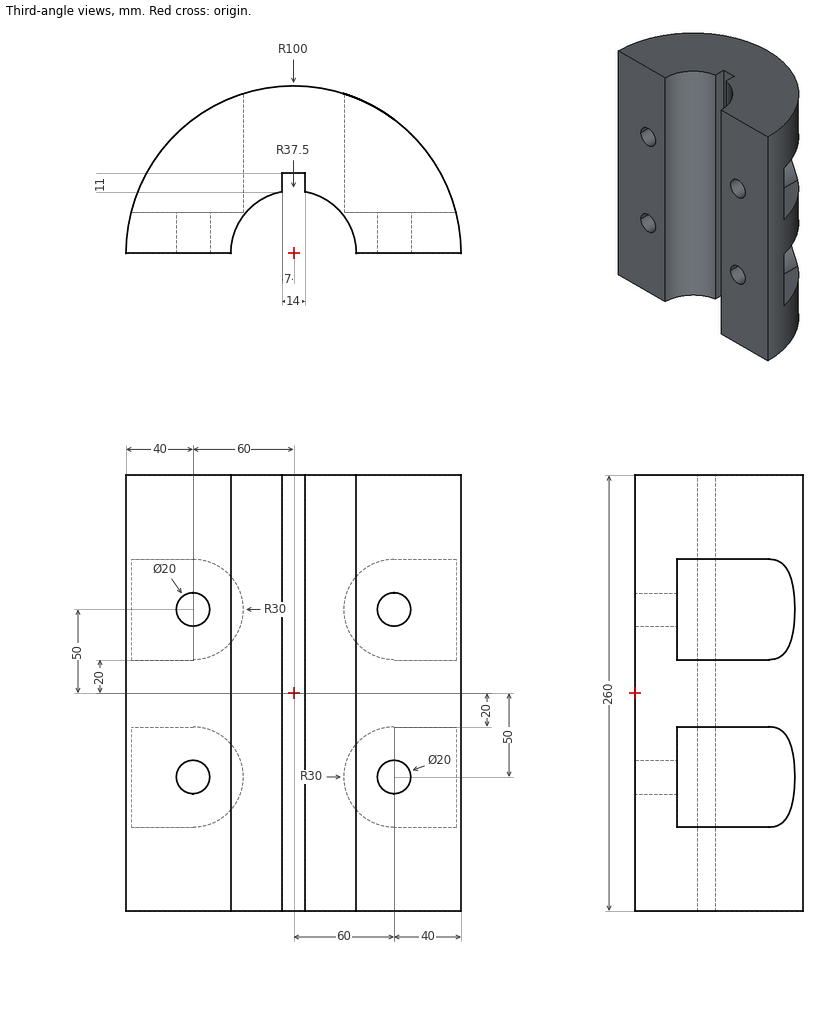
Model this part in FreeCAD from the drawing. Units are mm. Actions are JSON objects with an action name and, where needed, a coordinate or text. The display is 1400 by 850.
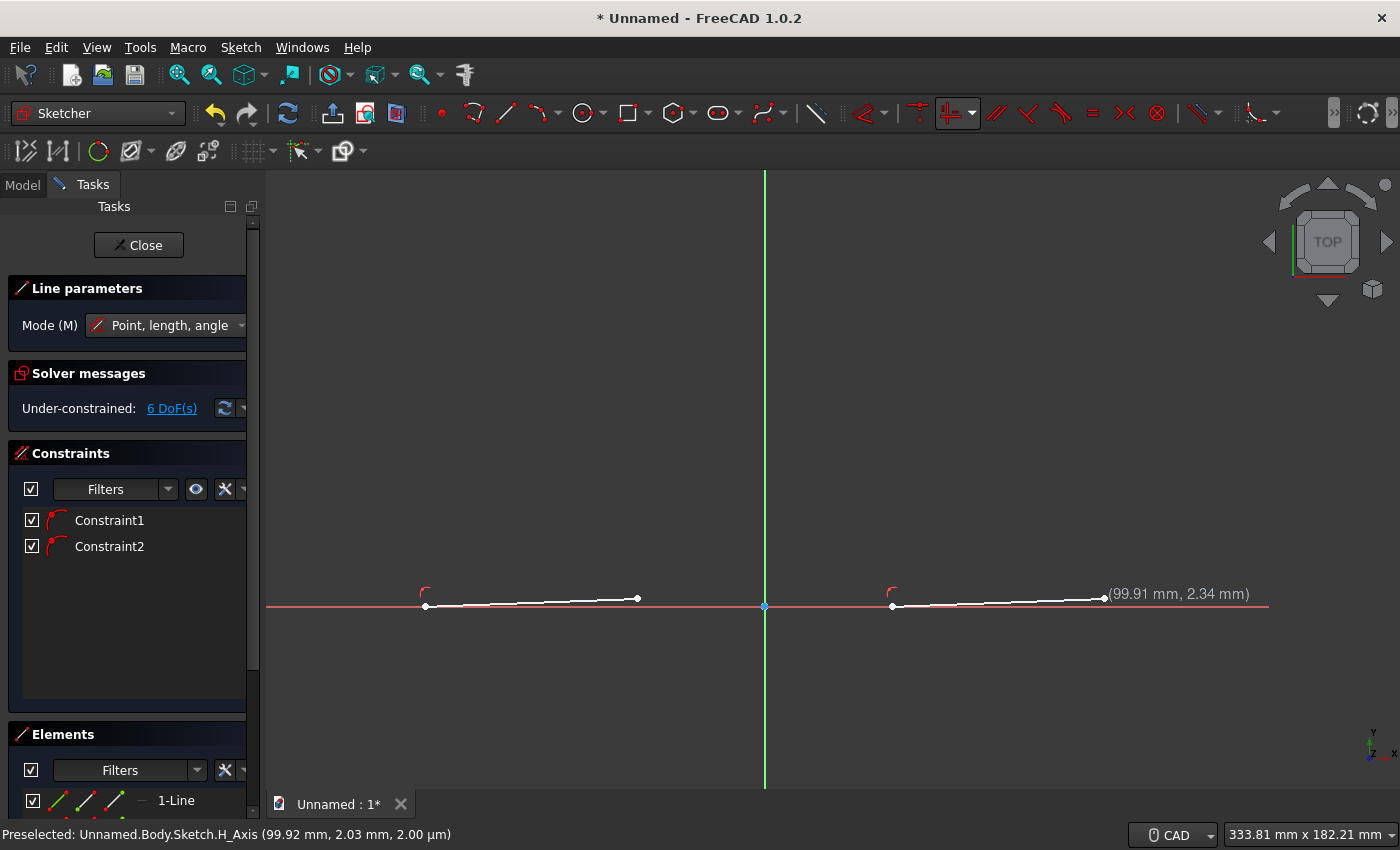
{"action": "left_click", "coordinate": [538, 114]}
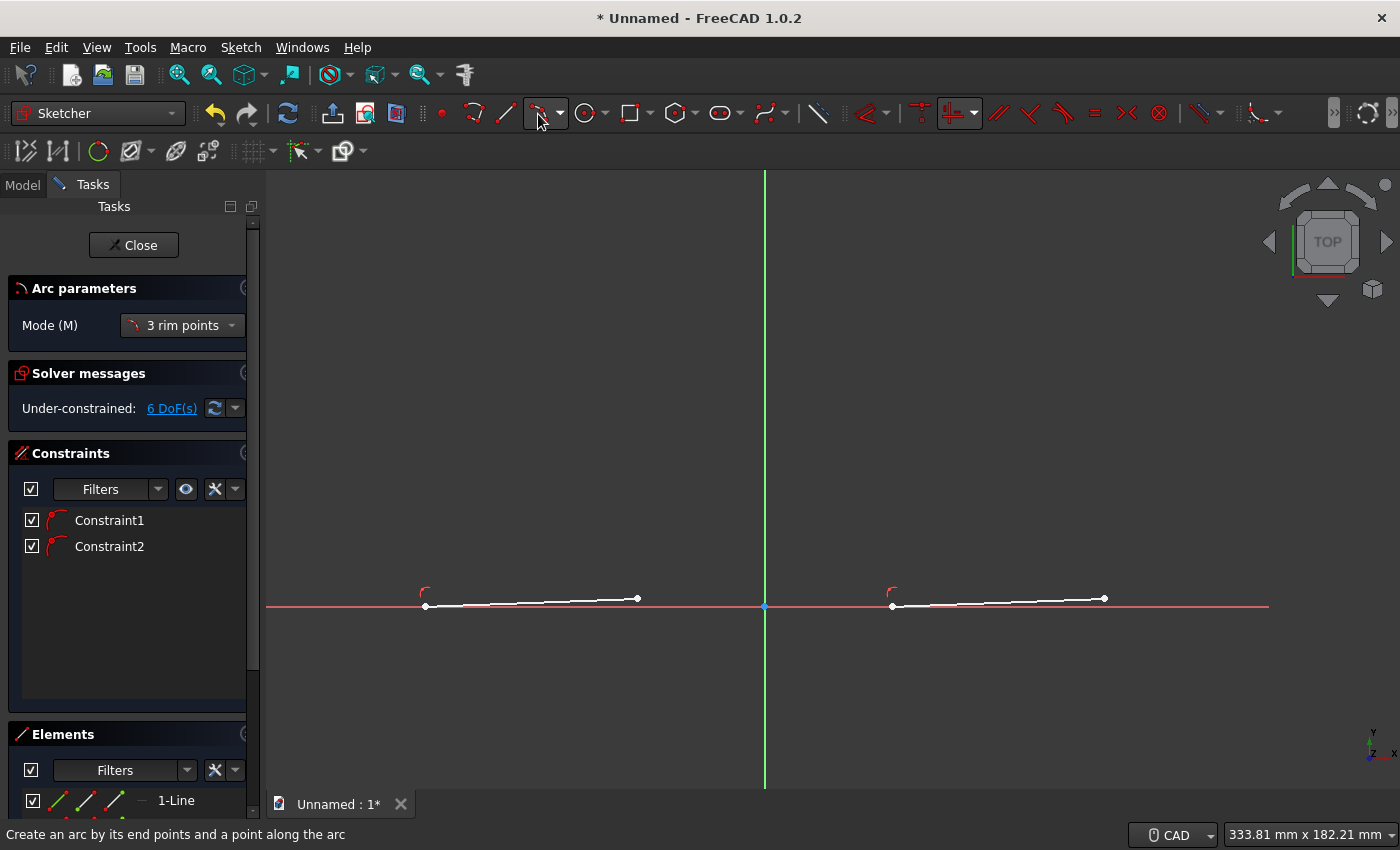
{"action": "left_click", "coordinate": [637, 599]}
{"action": "left_click", "coordinate": [892, 607]}
{"action": "left_click", "coordinate": [804, 486]}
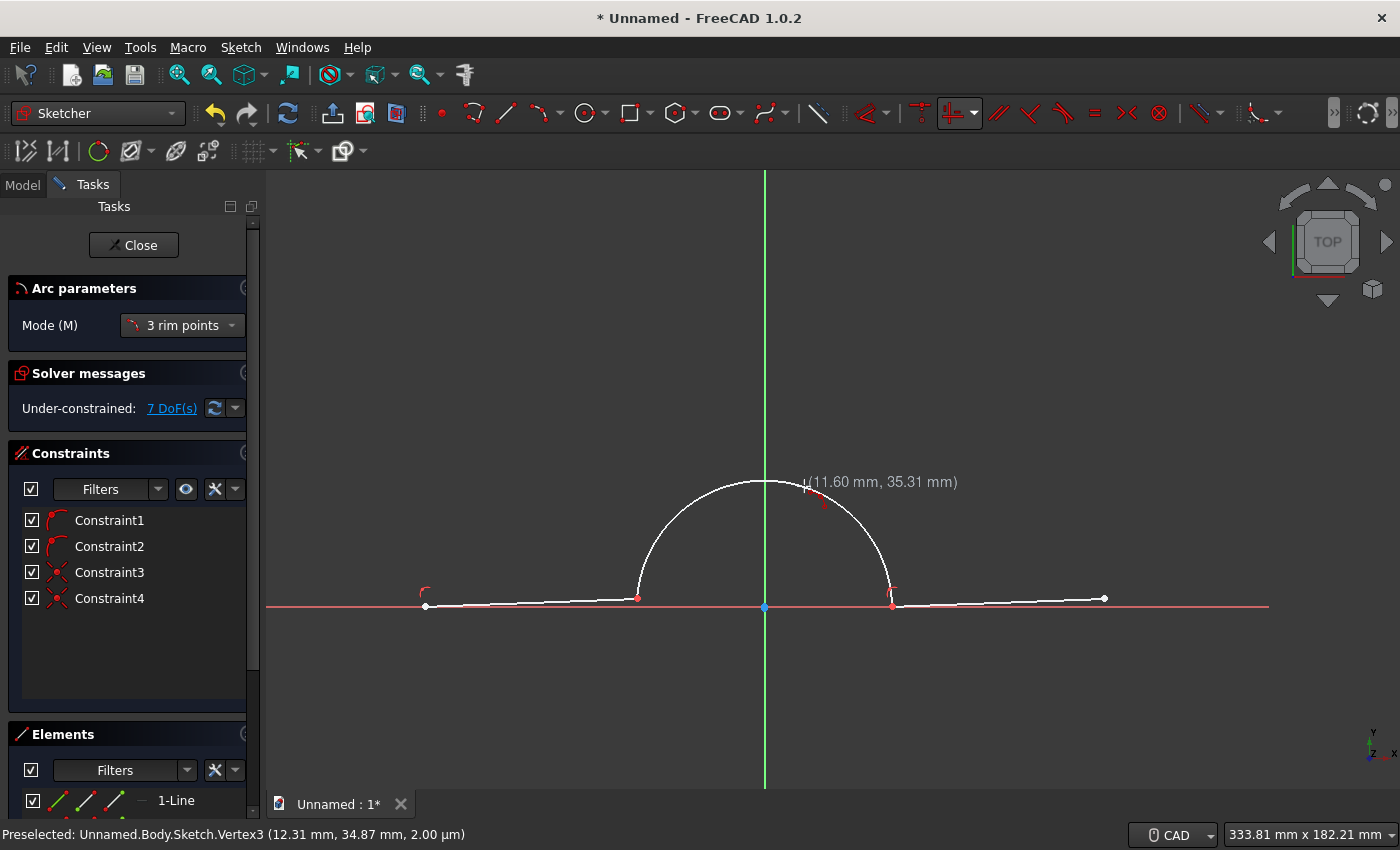
{"action": "left_click", "coordinate": [1104, 599]}
{"action": "left_click", "coordinate": [425, 607]}
{"action": "left_click", "coordinate": [870, 284]}
{"action": "key", "text": "Escape"}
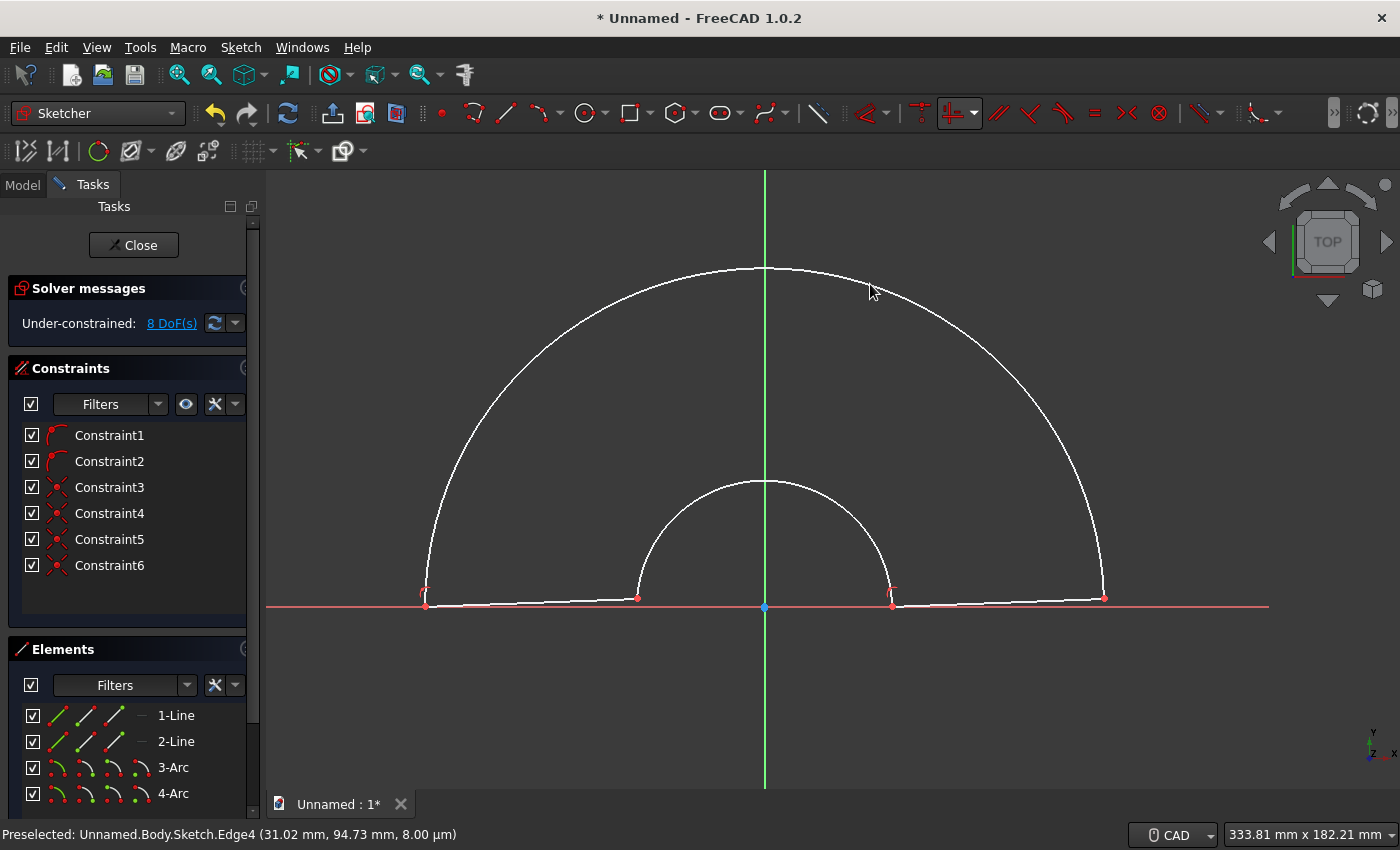
{"action": "left_click", "coordinate": [489, 605]}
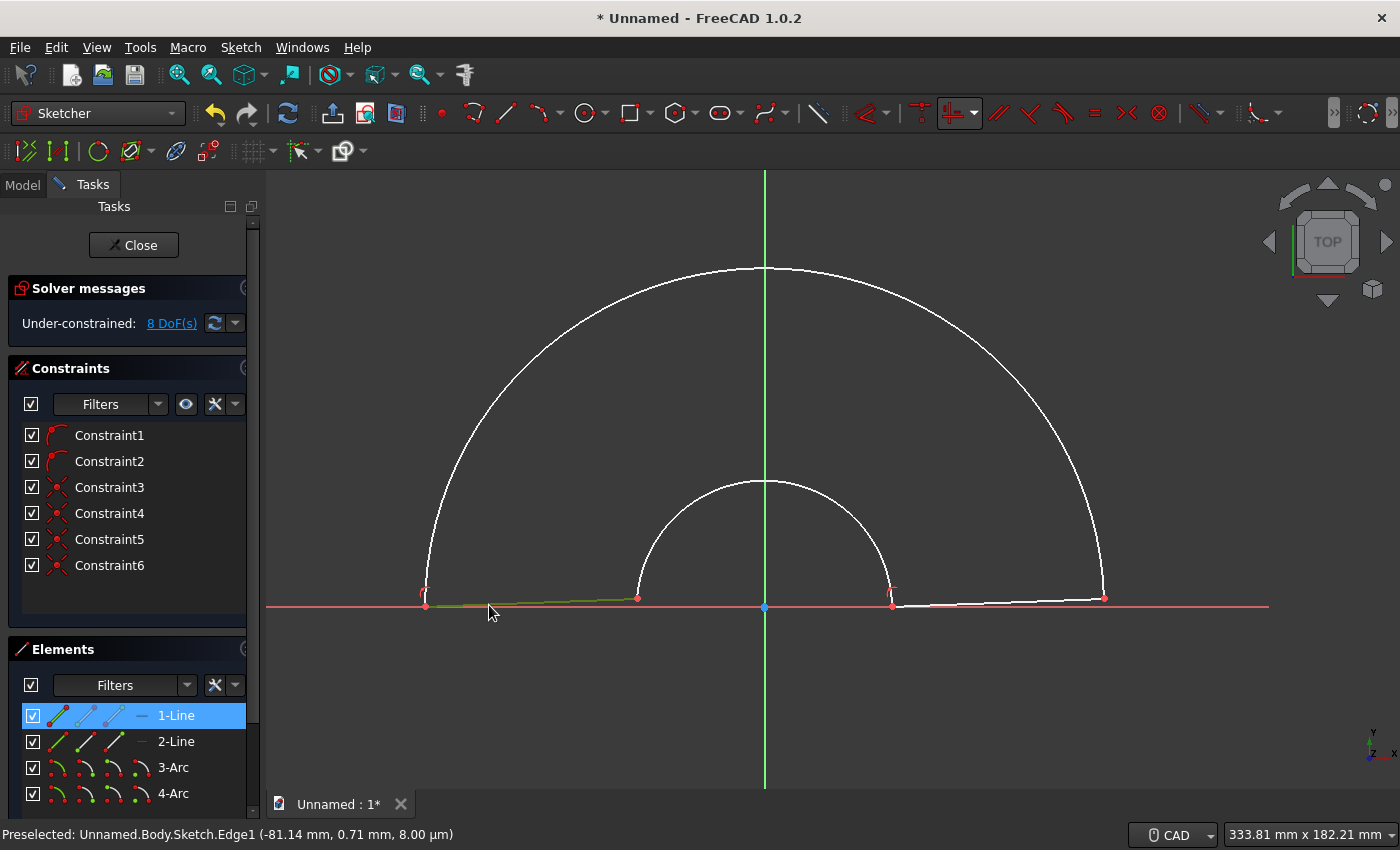
{"action": "key", "text": "h"}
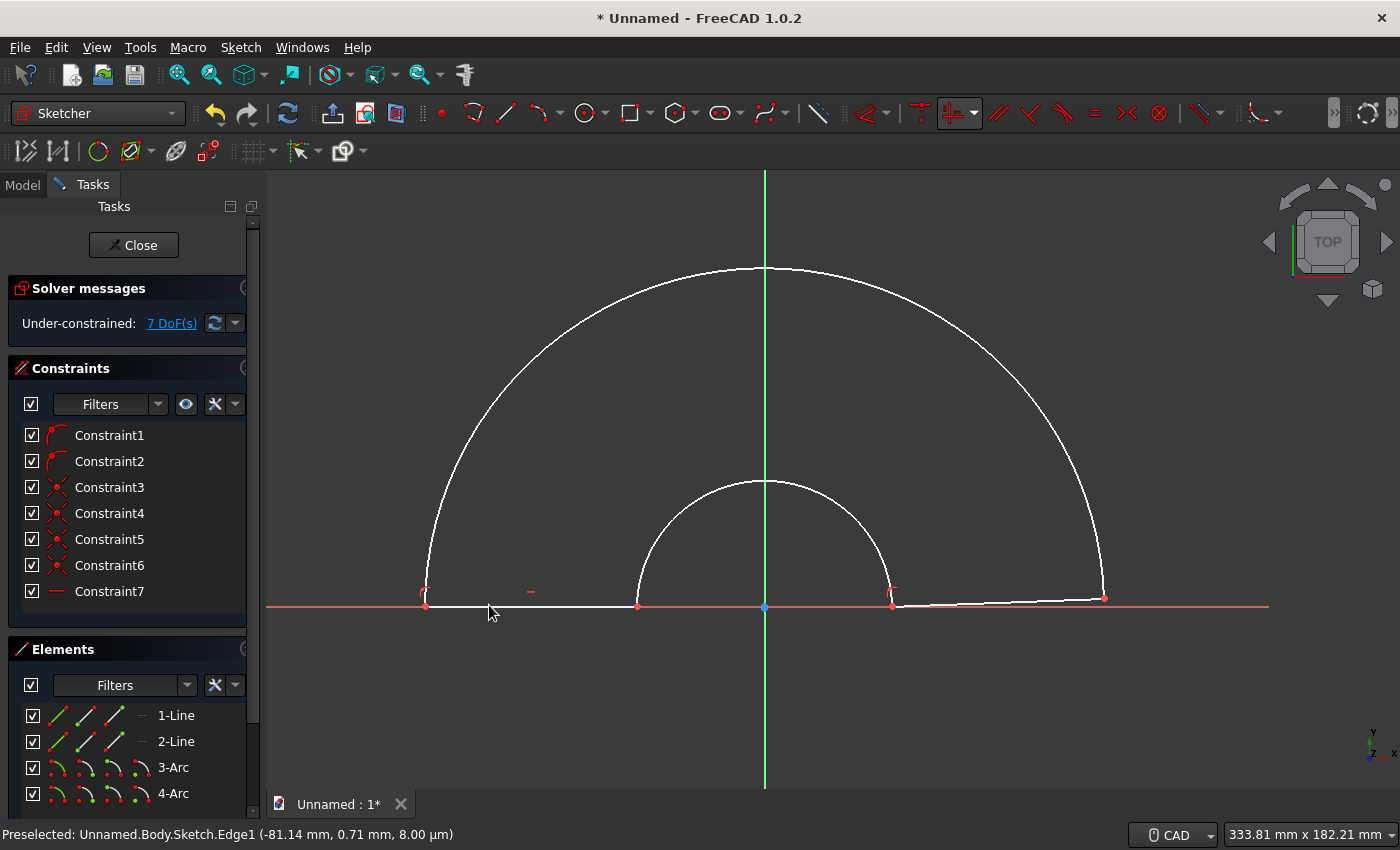
{"action": "left_click", "coordinate": [956, 605]}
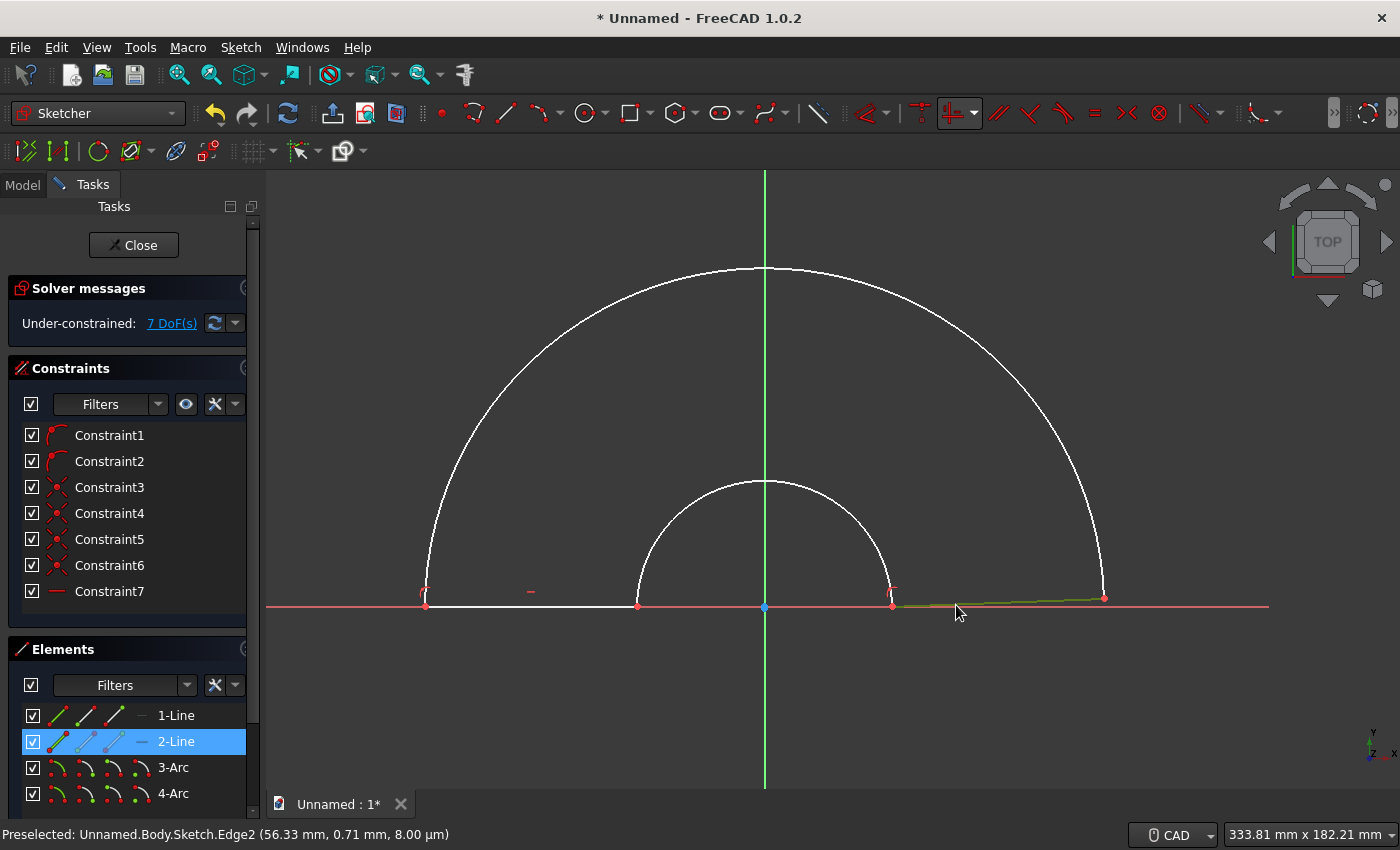
{"action": "left_click", "coordinate": [976, 114]}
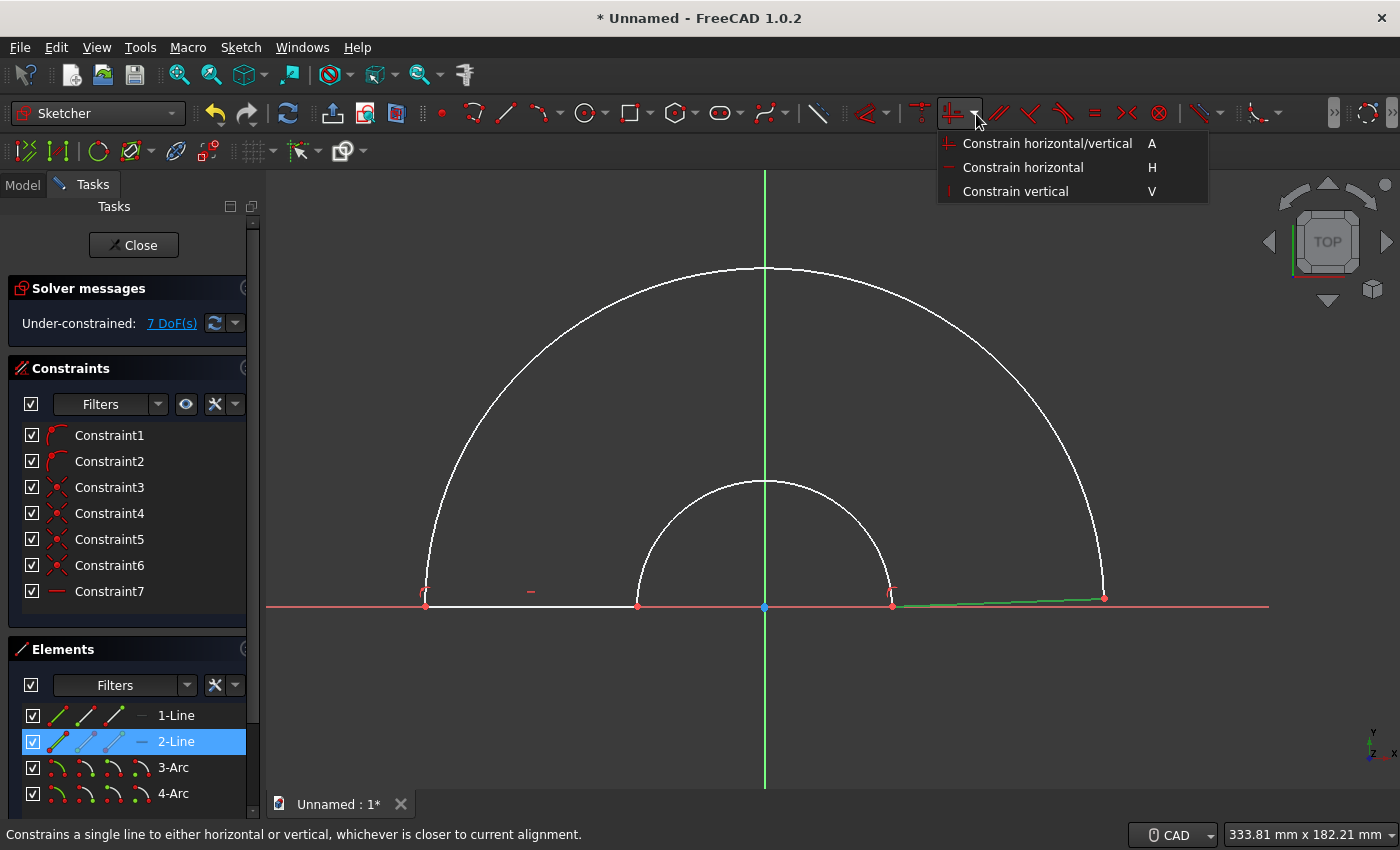
{"action": "left_click", "coordinate": [1073, 167]}